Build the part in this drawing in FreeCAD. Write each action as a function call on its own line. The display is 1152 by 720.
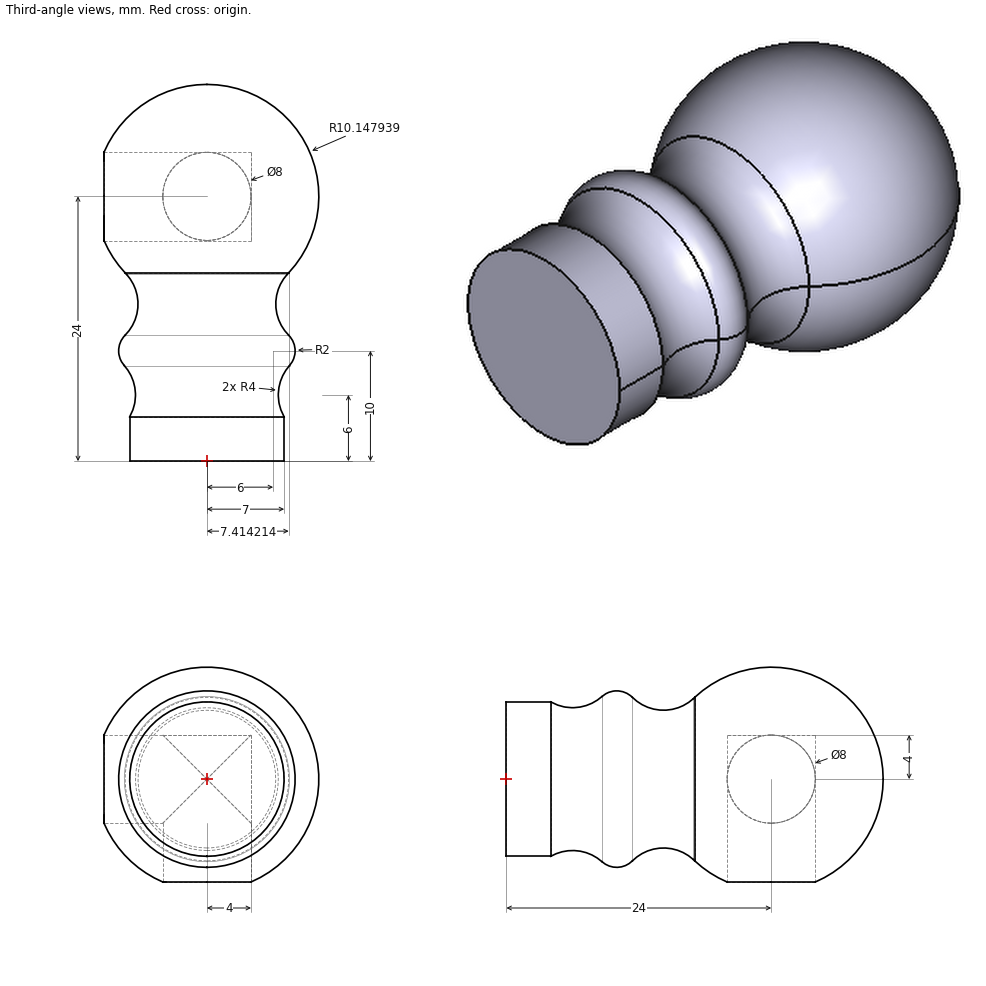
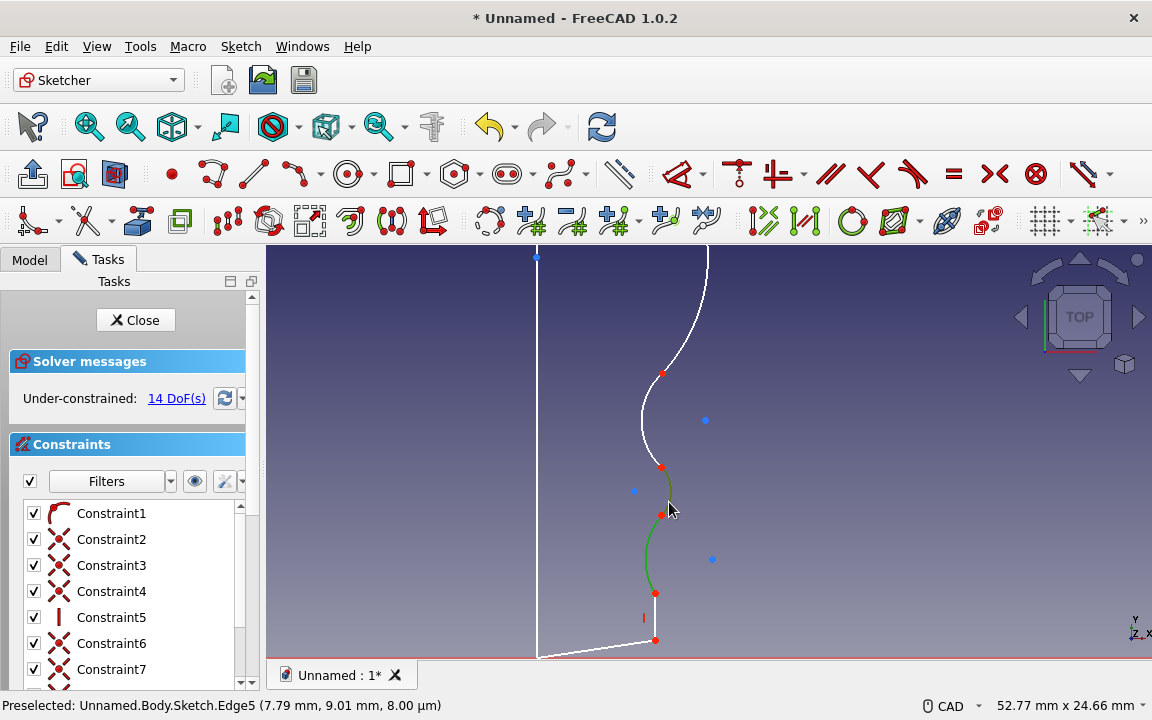
click(913, 174)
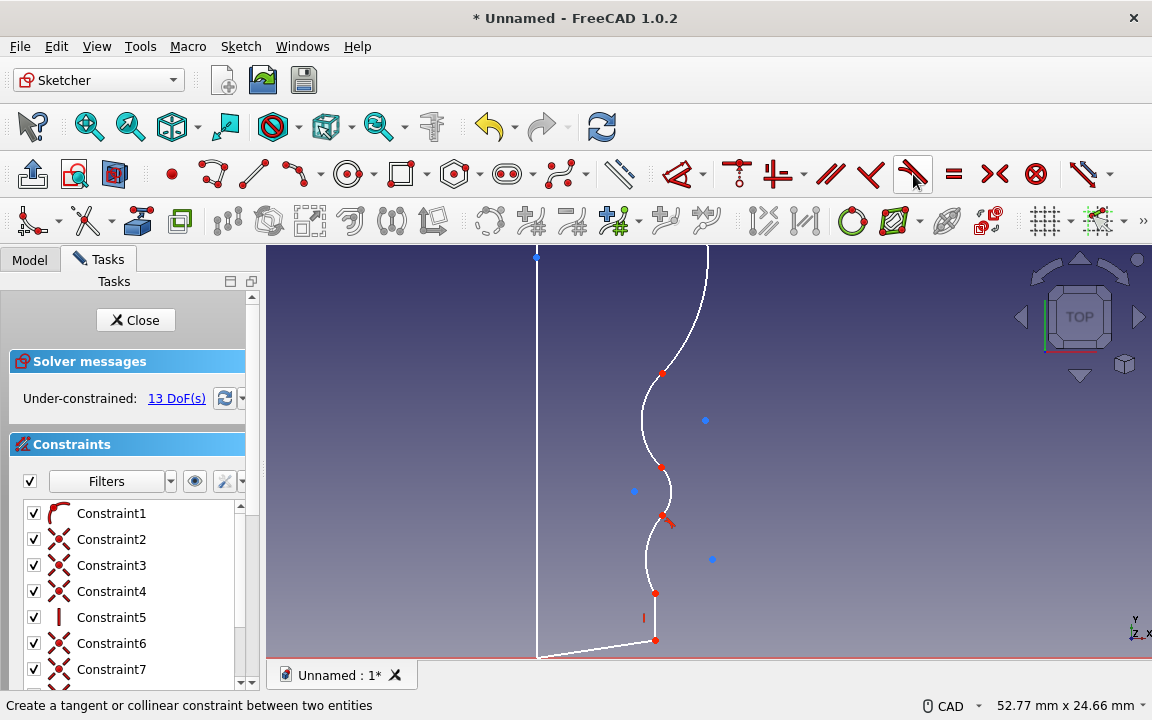
click(670, 502)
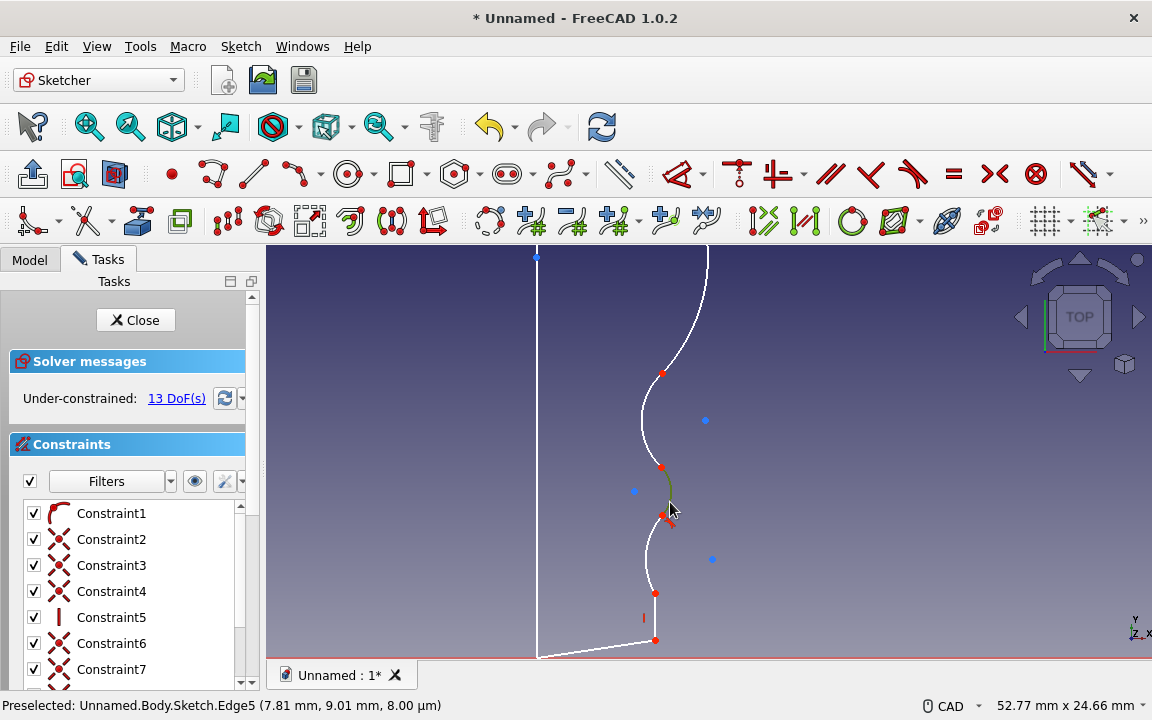
click(645, 399)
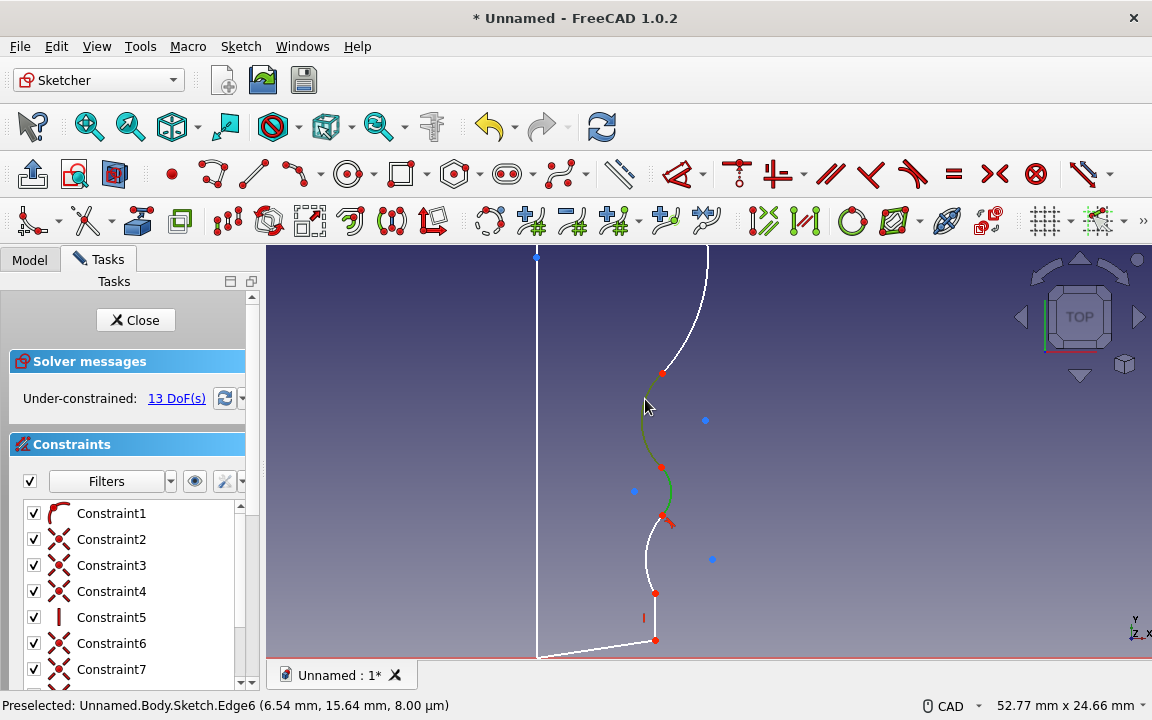
click(913, 174)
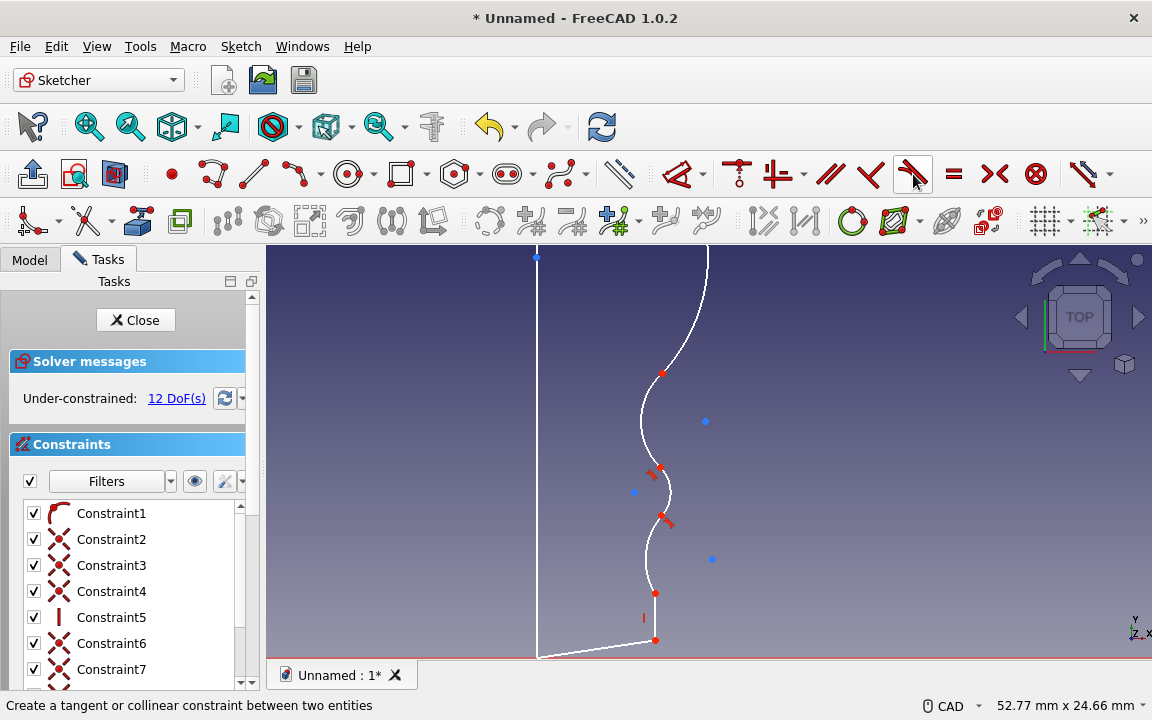
scroll(661, 518, down, 4)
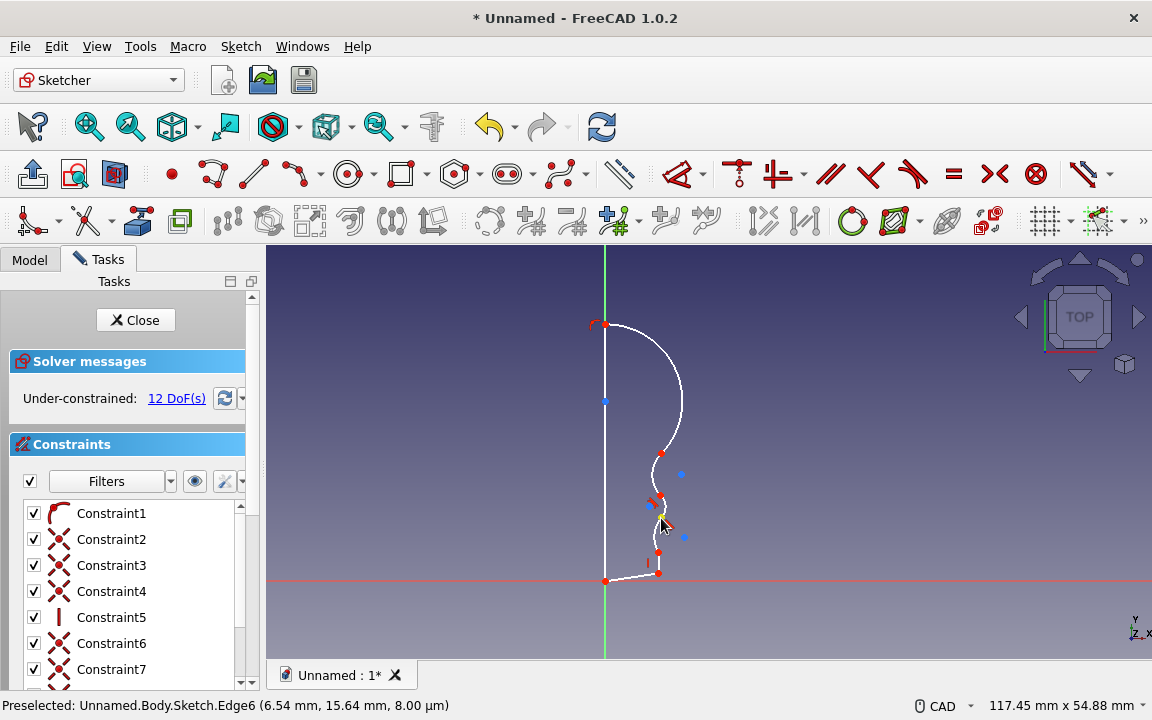
scroll(643, 576, up, 5)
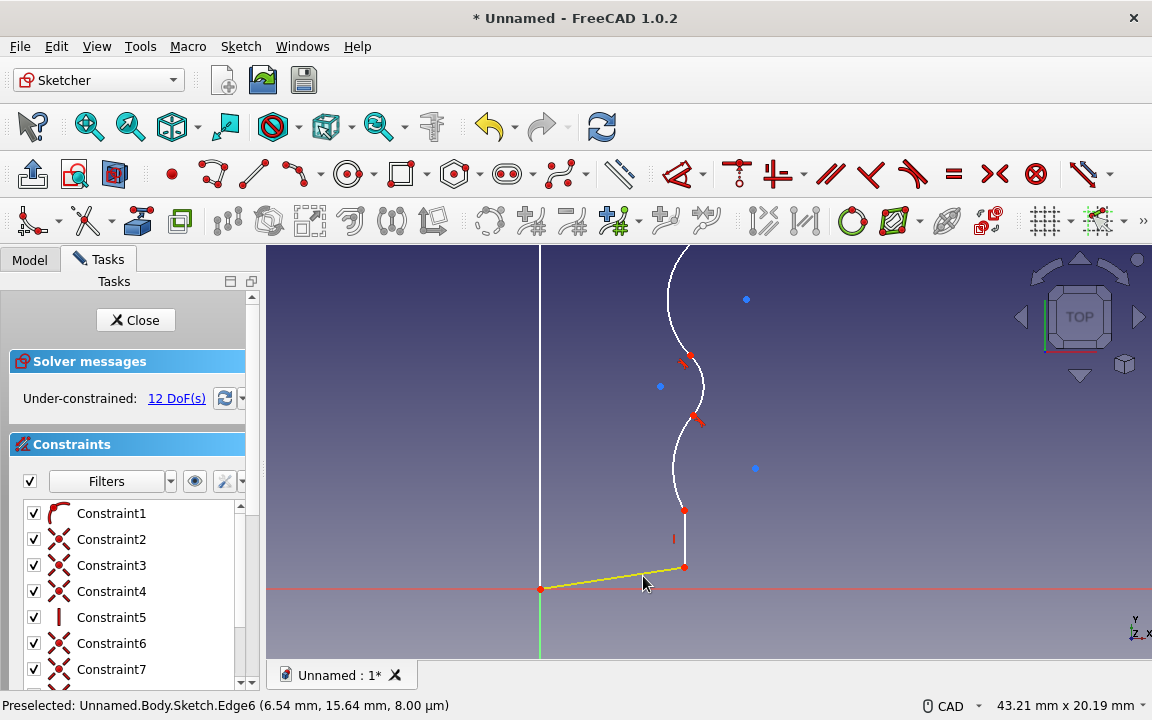
click(641, 574)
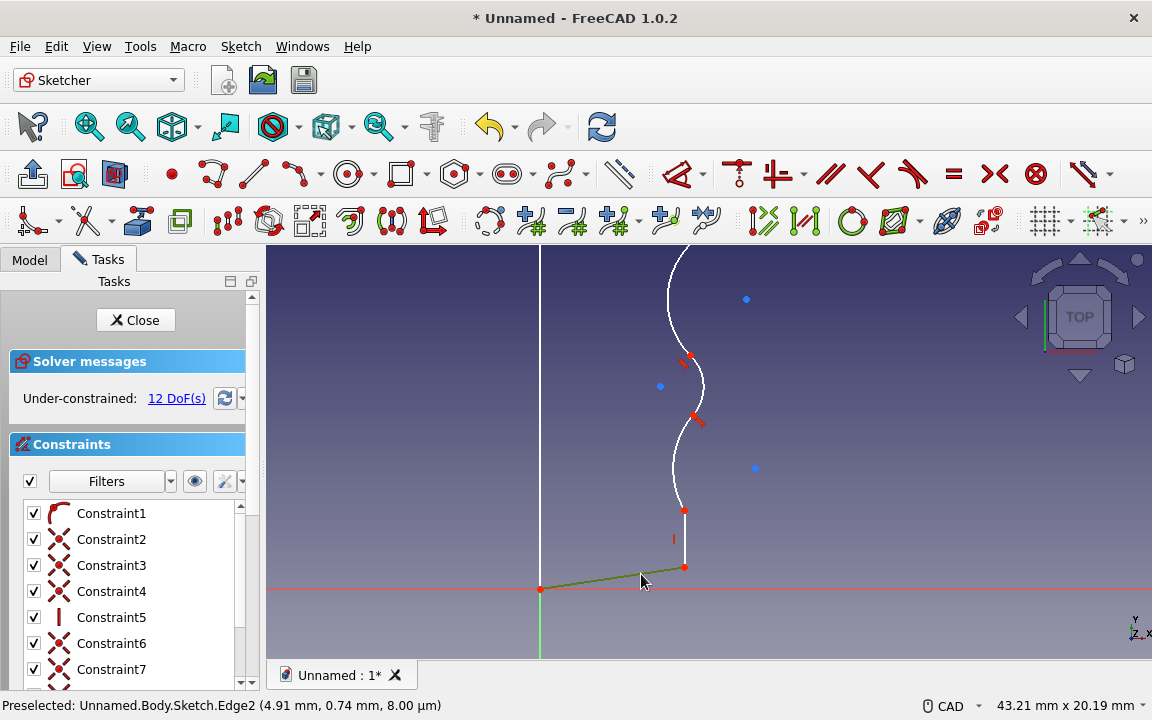
click(804, 174)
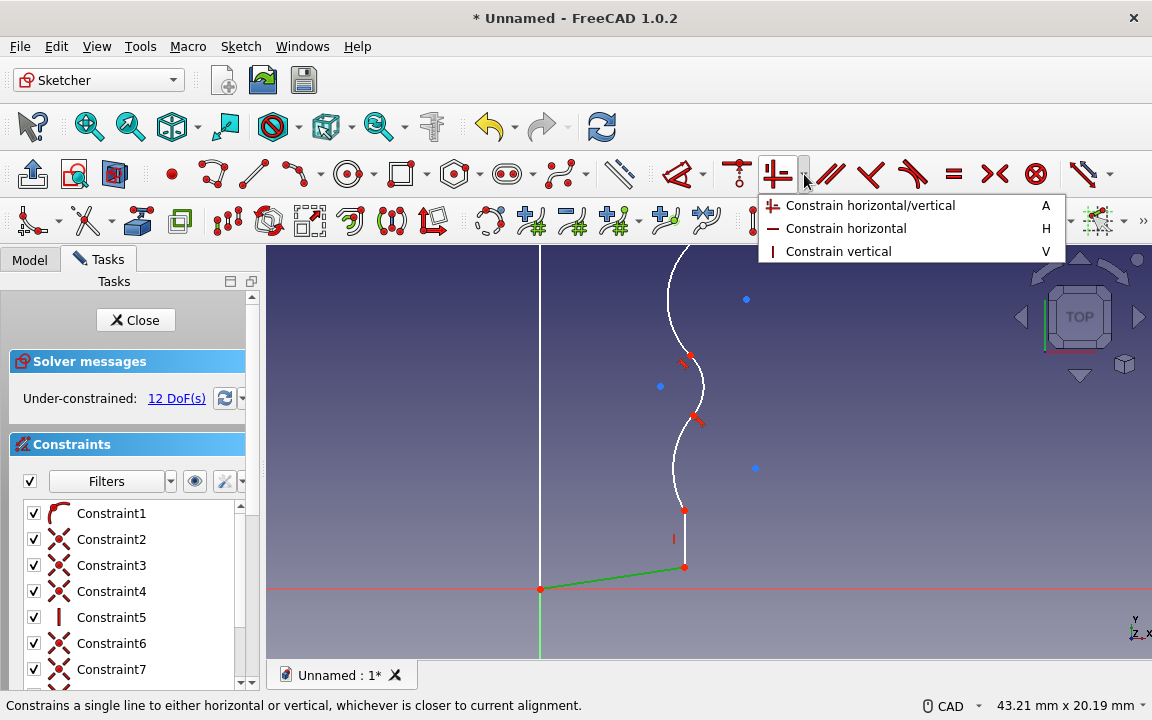
click(912, 228)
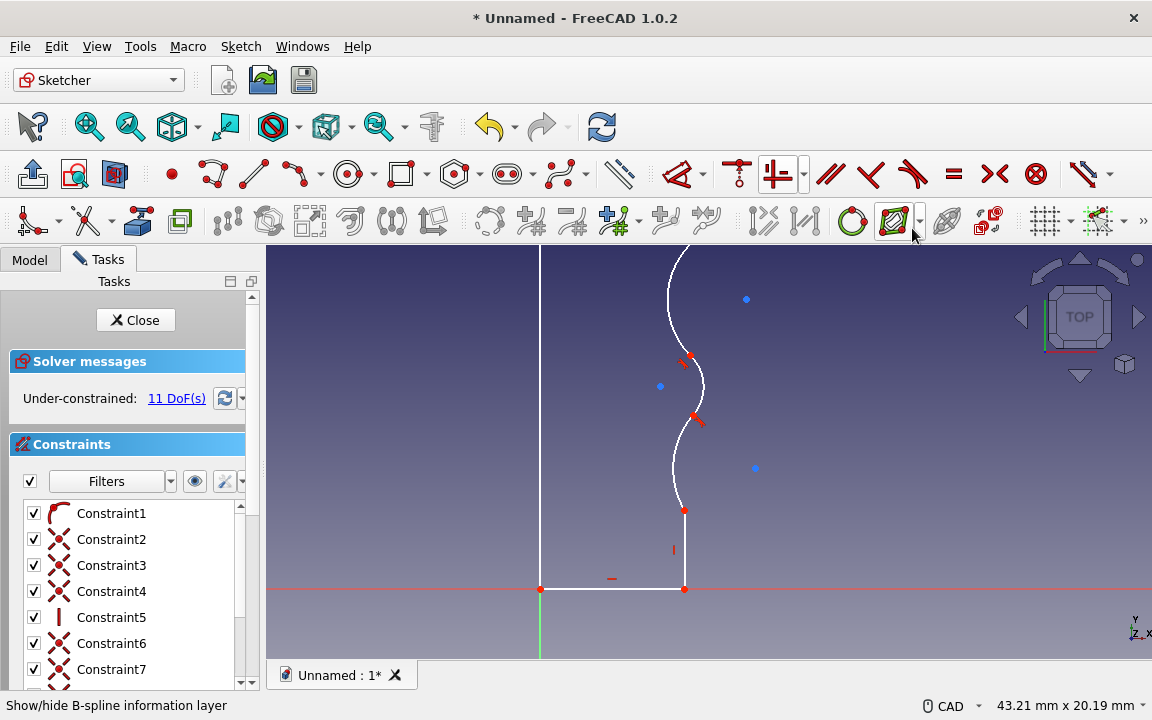
click(678, 442)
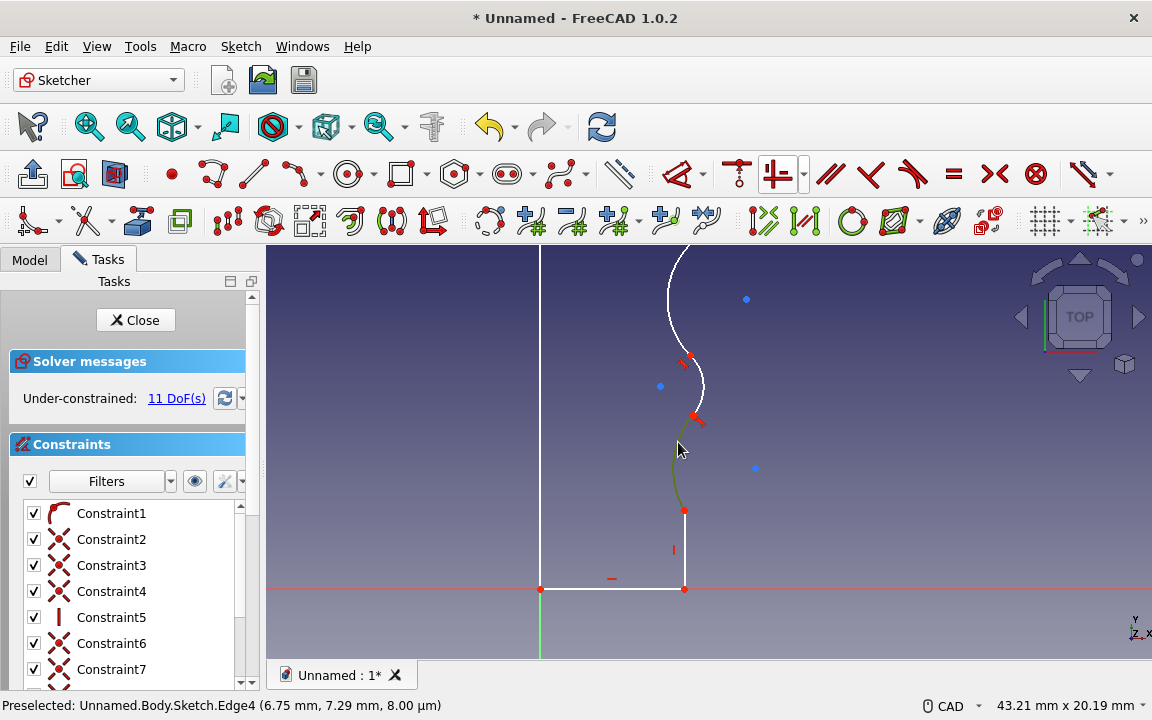
click(671, 323)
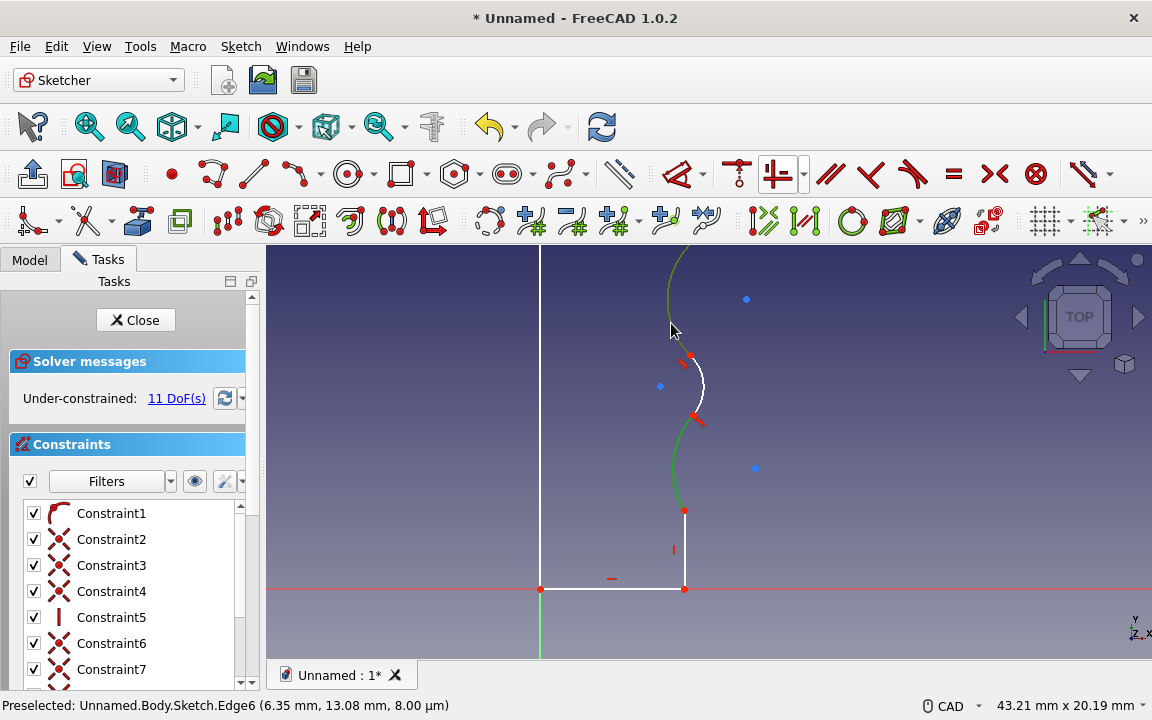
click(954, 174)